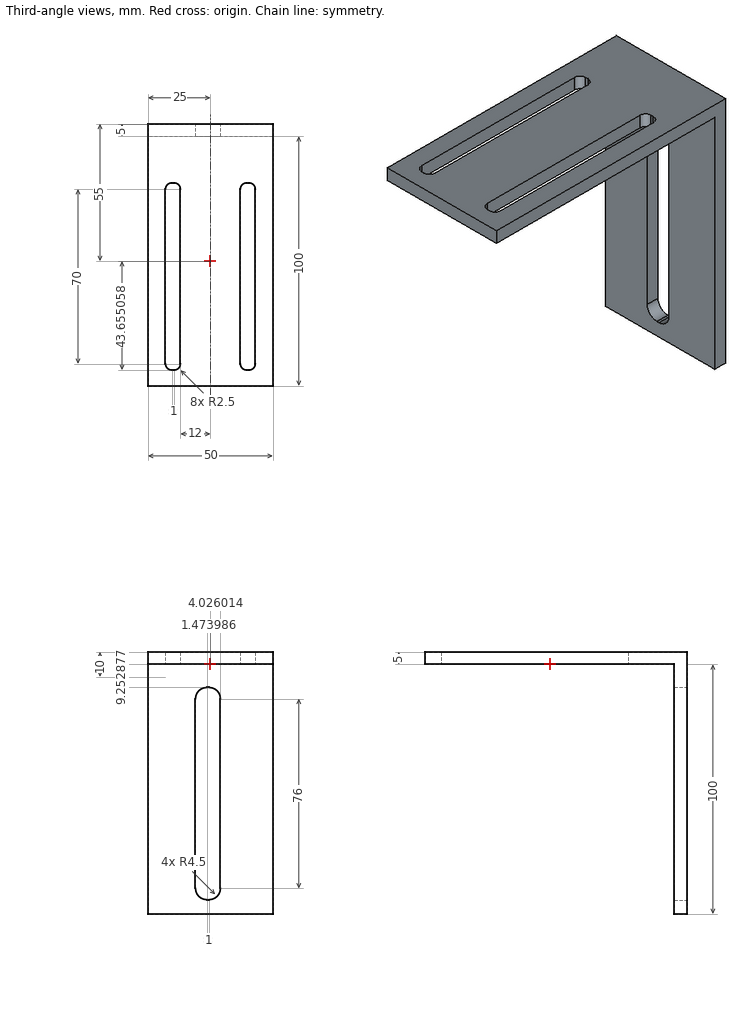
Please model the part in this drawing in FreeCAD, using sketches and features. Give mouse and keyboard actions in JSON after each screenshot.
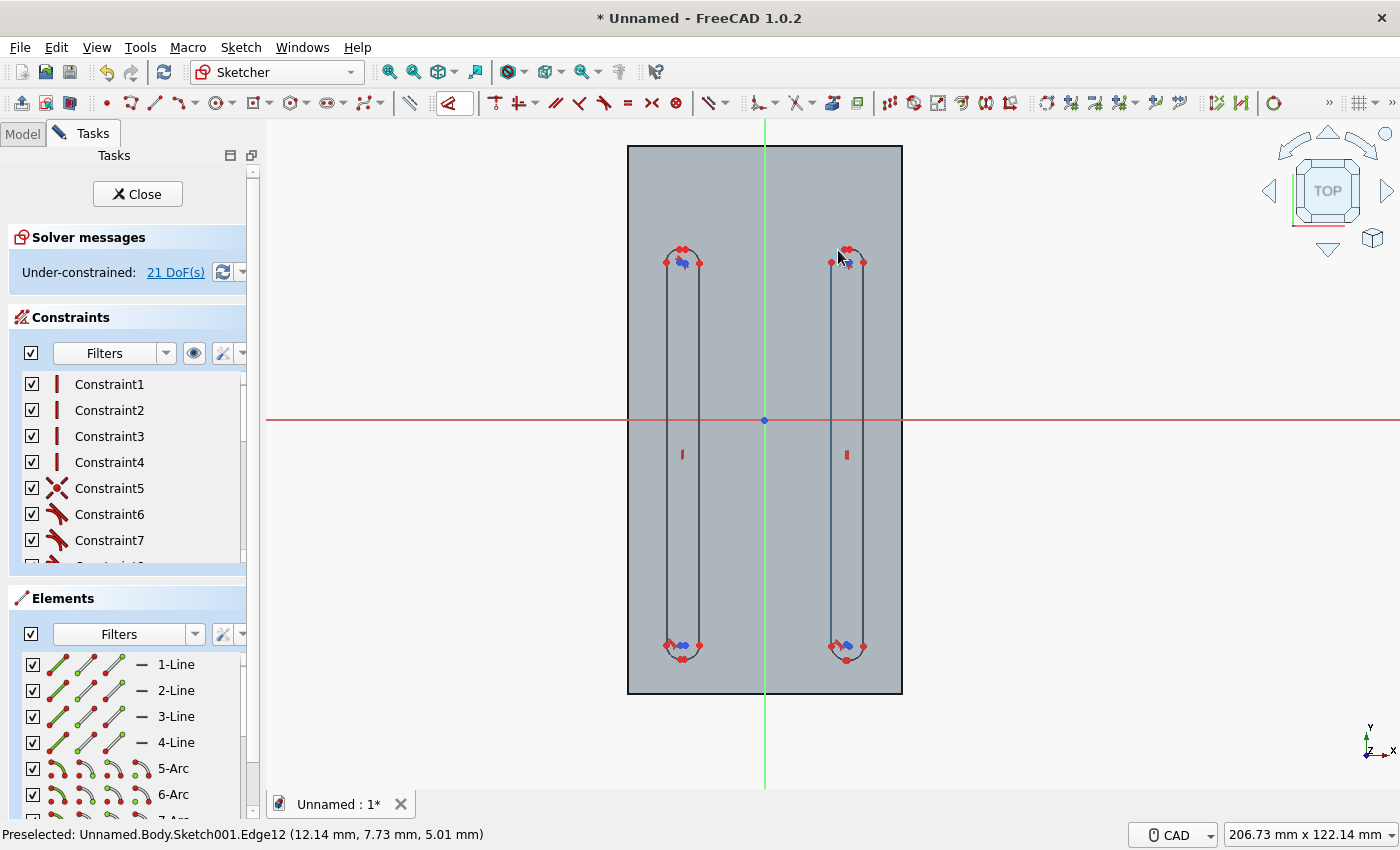
{"action": "scroll", "coordinate": [833, 653], "scroll_direction": "up", "scroll_amount": 5}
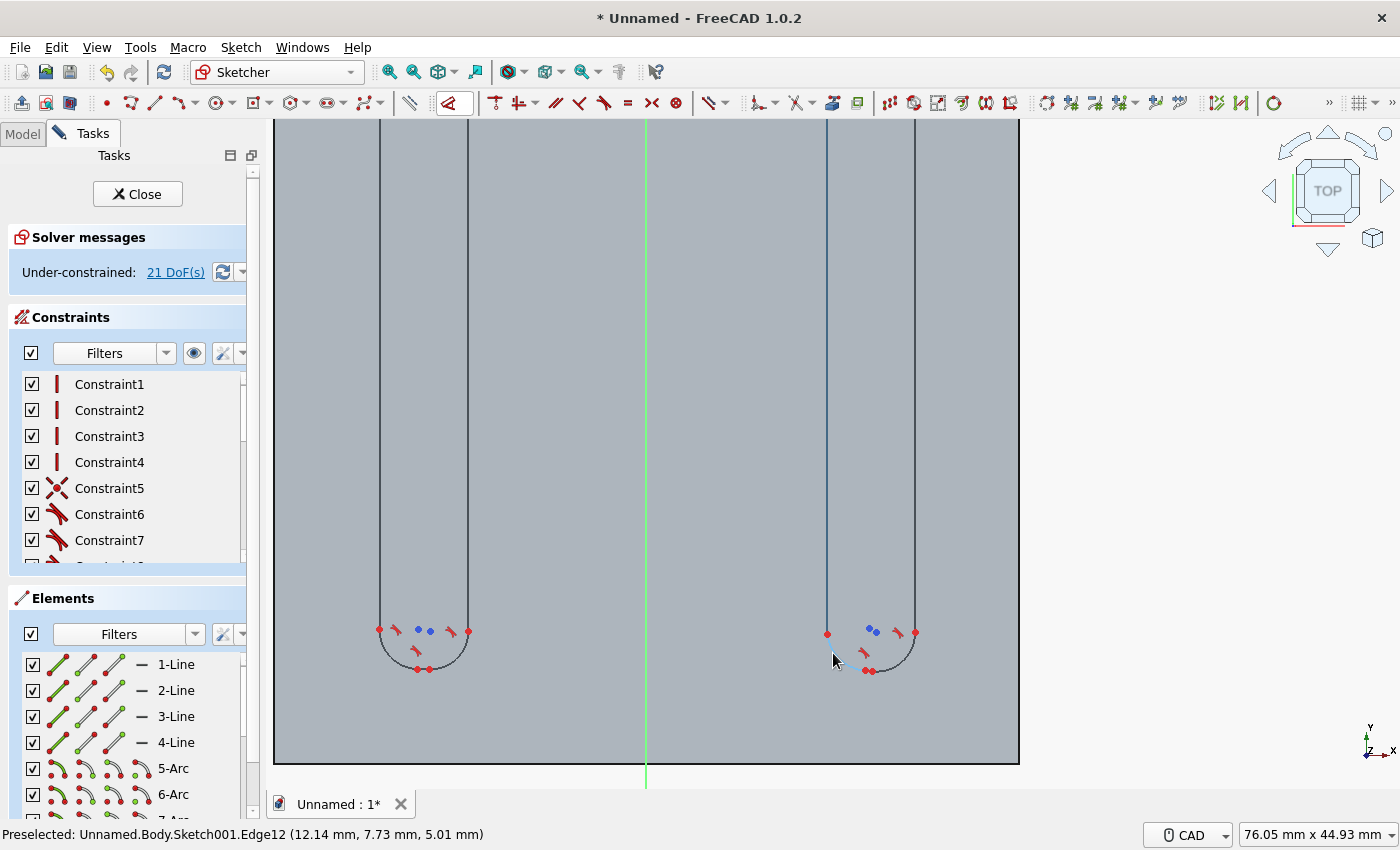
{"action": "left_click", "coordinate": [833, 650]}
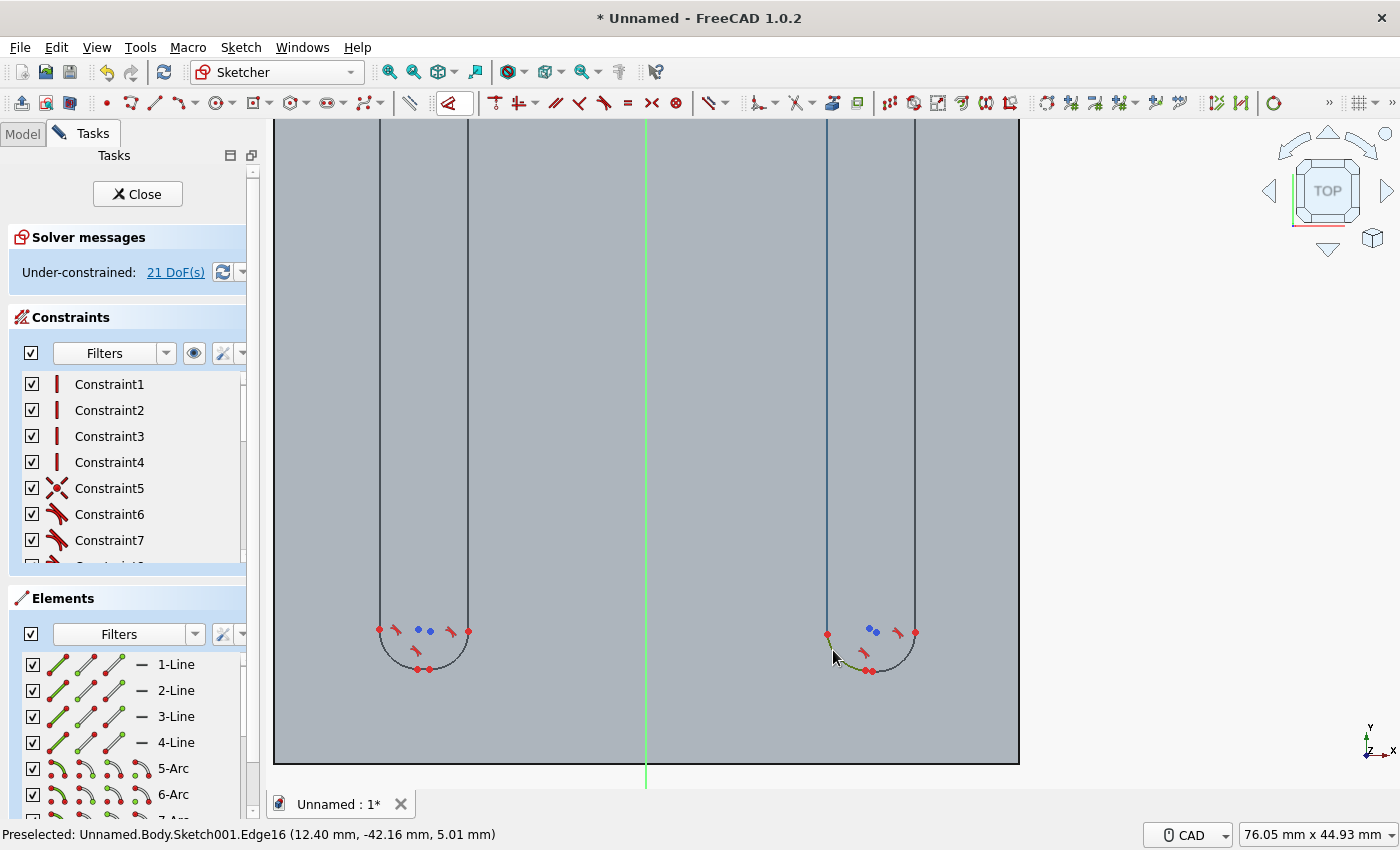
{"action": "key", "text": "t"}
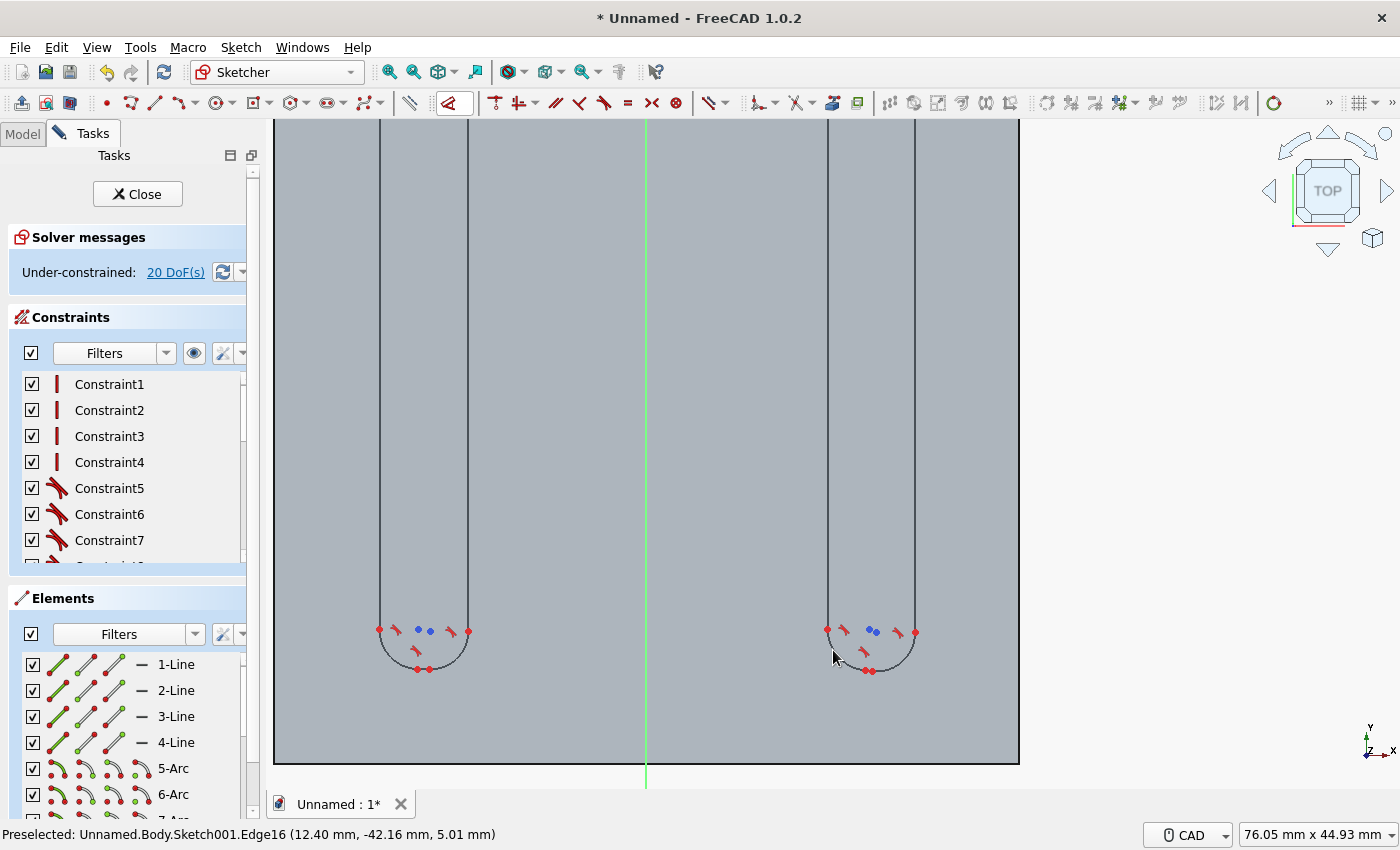
{"action": "scroll", "coordinate": [424, 669], "scroll_direction": "up", "scroll_amount": 5}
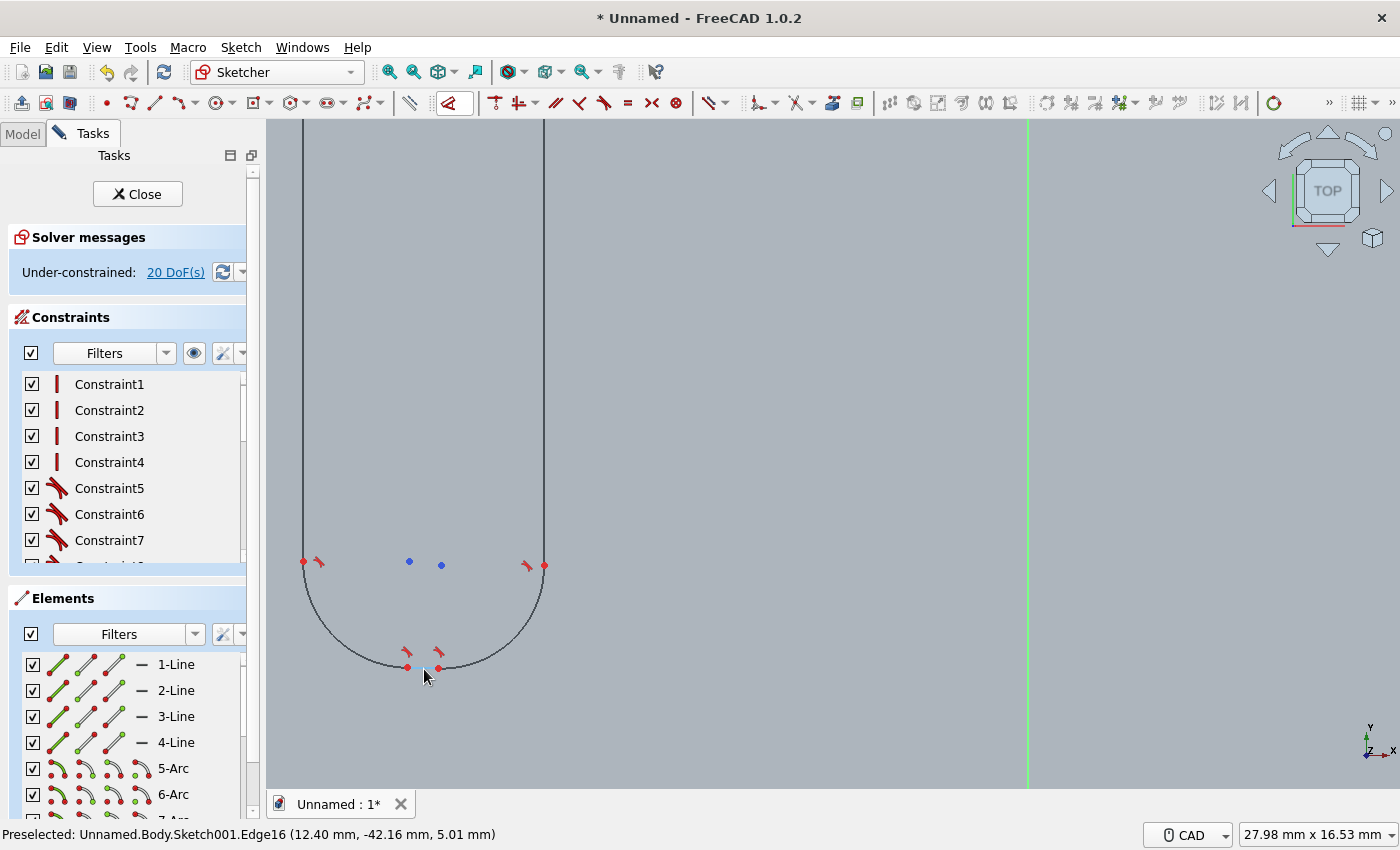
{"action": "left_click", "coordinate": [423, 668]}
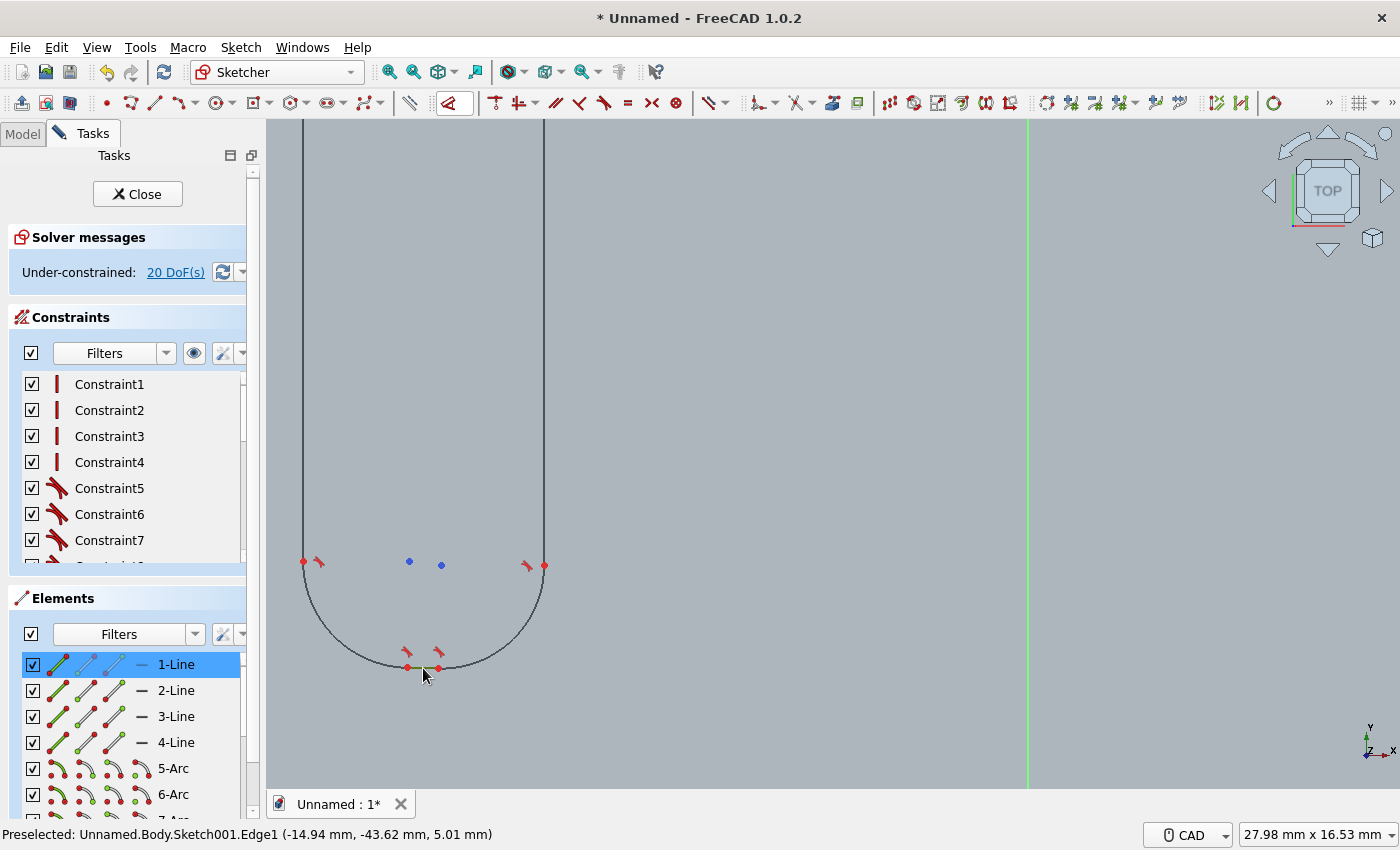
{"action": "key", "text": "h"}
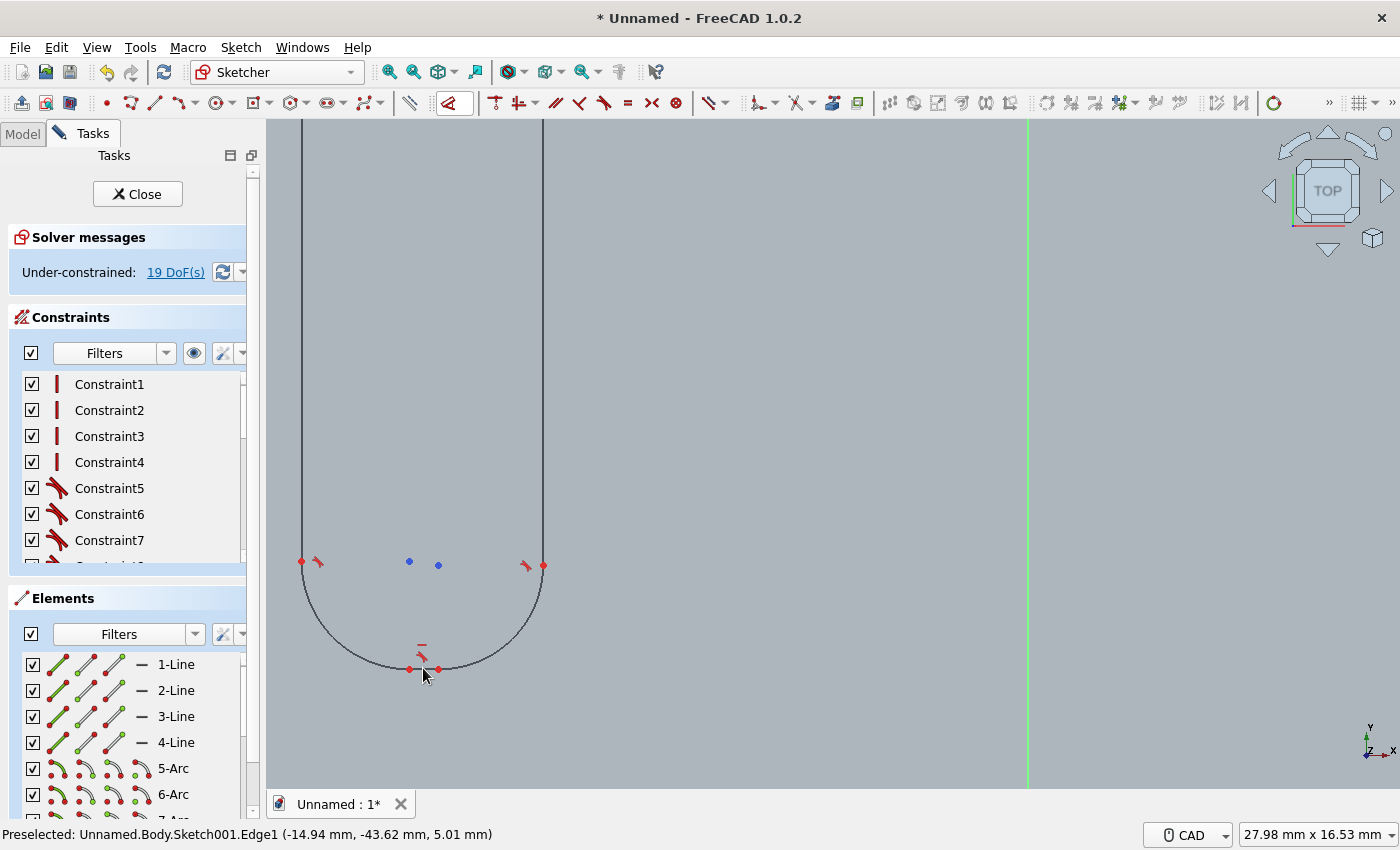
{"action": "scroll", "coordinate": [723, 658], "scroll_direction": "down", "scroll_amount": 10}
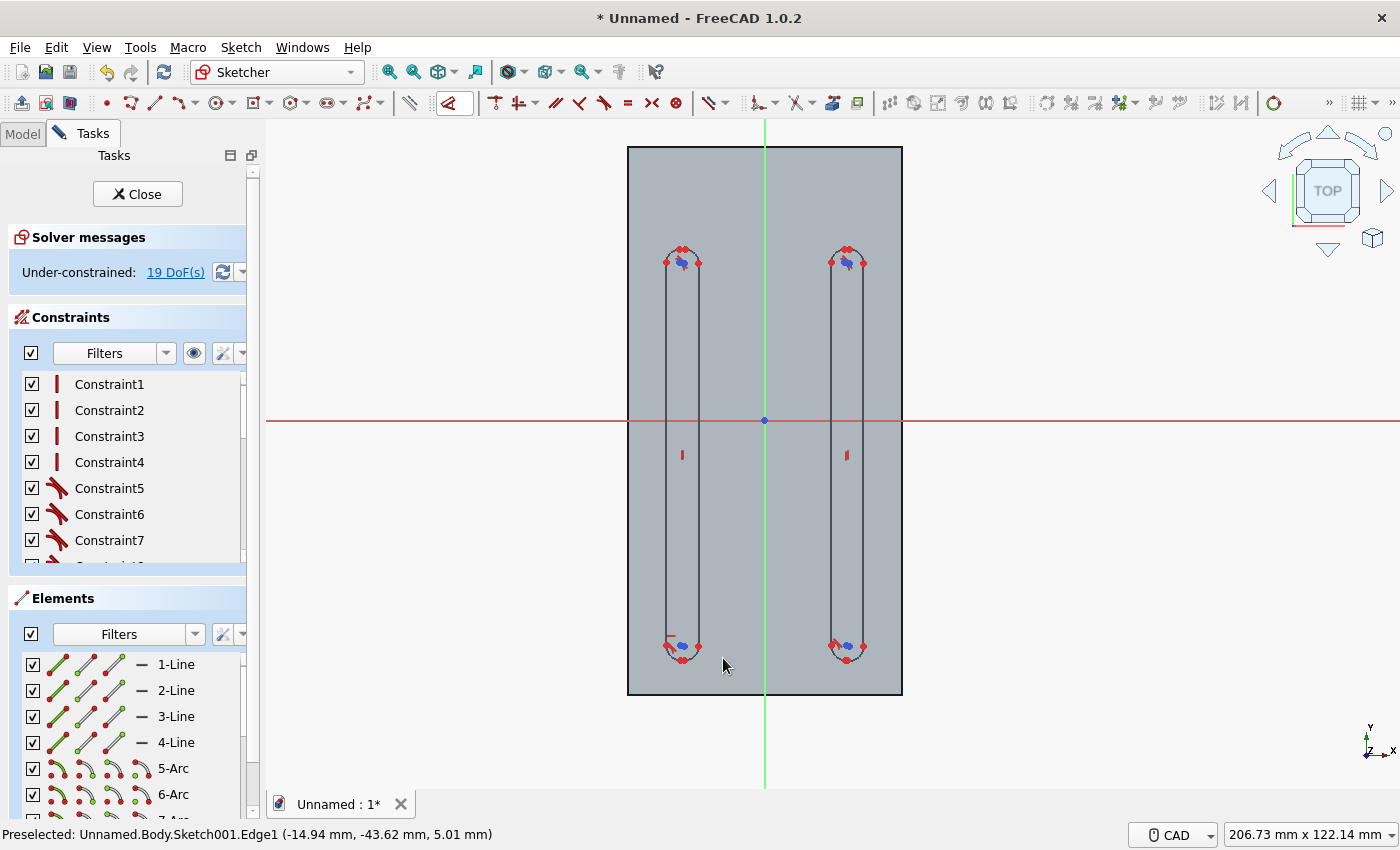
{"action": "scroll", "coordinate": [684, 250], "scroll_direction": "up", "scroll_amount": 11}